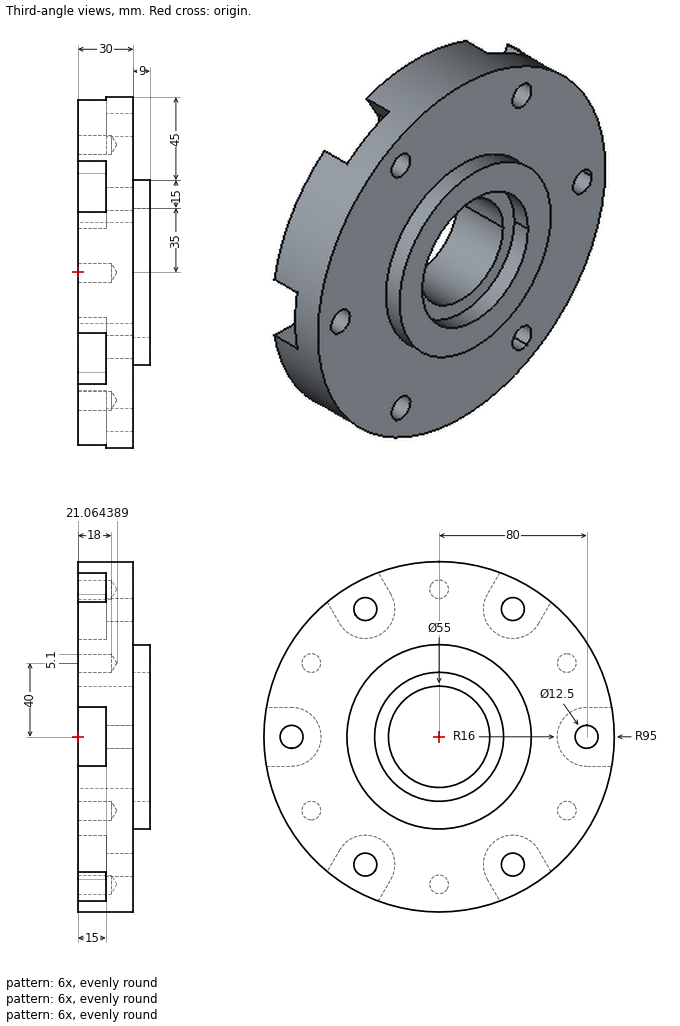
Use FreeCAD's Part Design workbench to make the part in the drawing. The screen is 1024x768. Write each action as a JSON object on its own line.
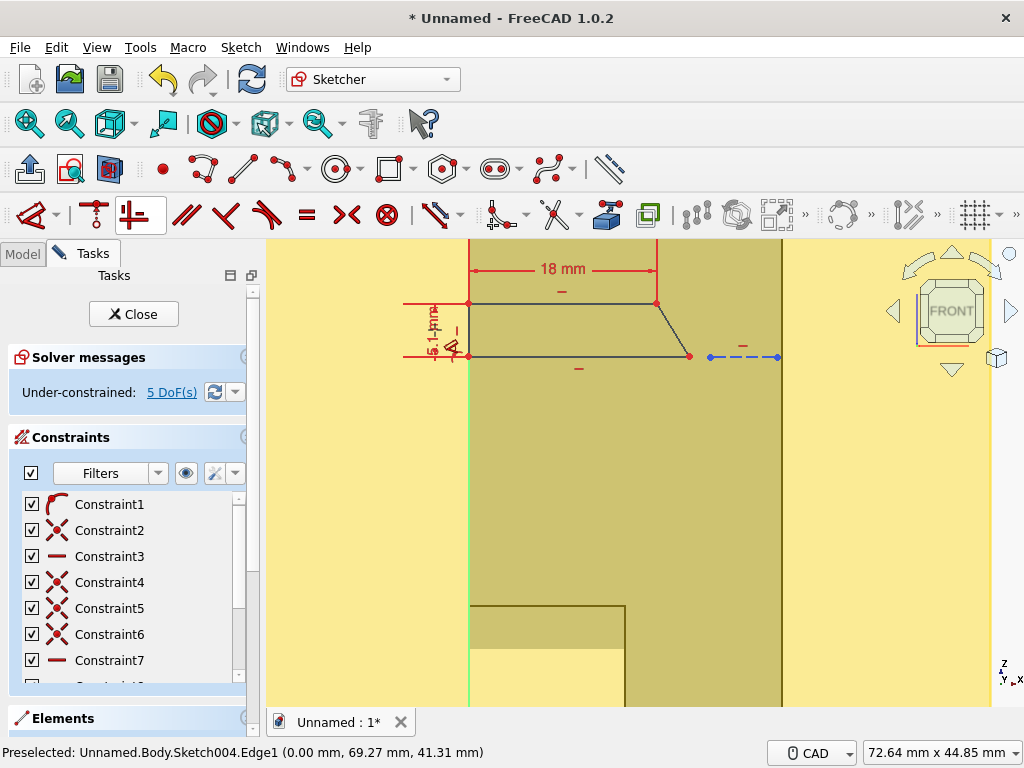
{"action": "left_click", "coordinate": [469, 357]}
{"action": "left_click", "coordinate": [435, 518]}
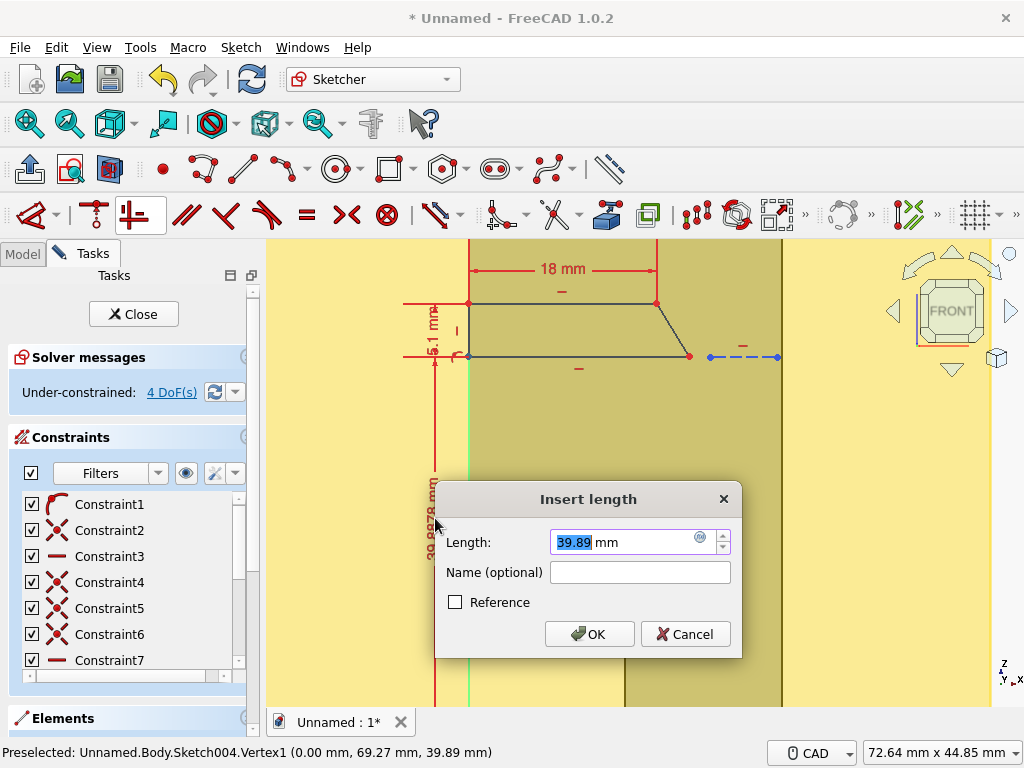
{"action": "type", "text": "40"}
{"action": "key", "text": "Return"}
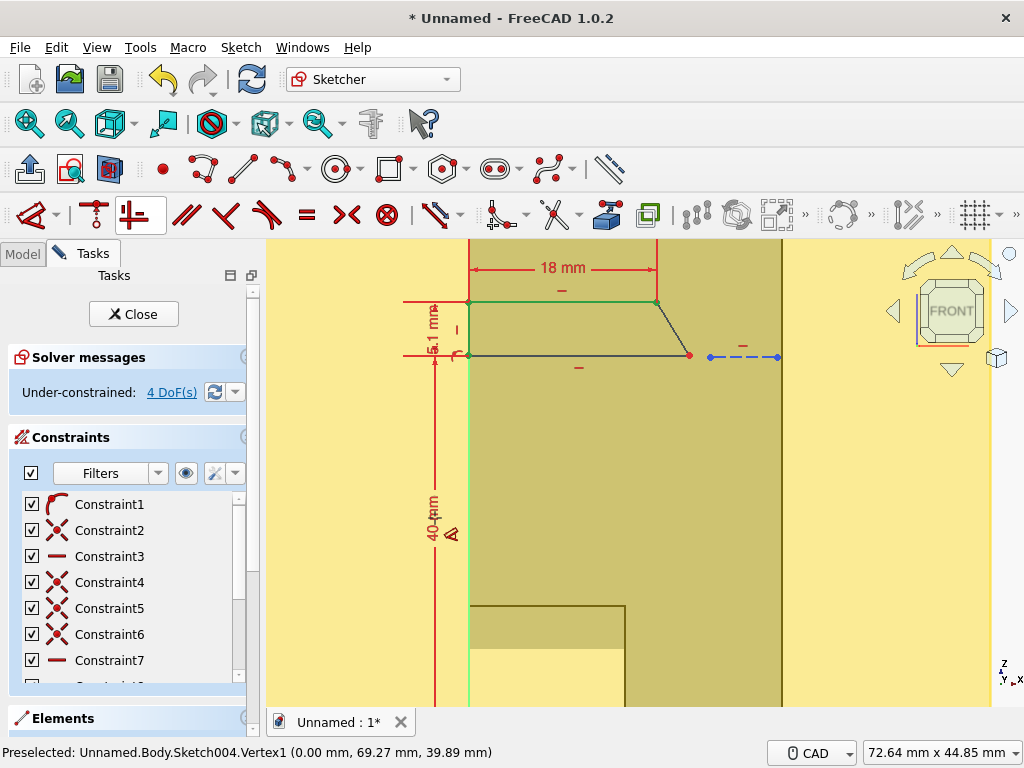
{"action": "left_click", "coordinate": [710, 357]}
{"action": "left_click", "coordinate": [435, 444]}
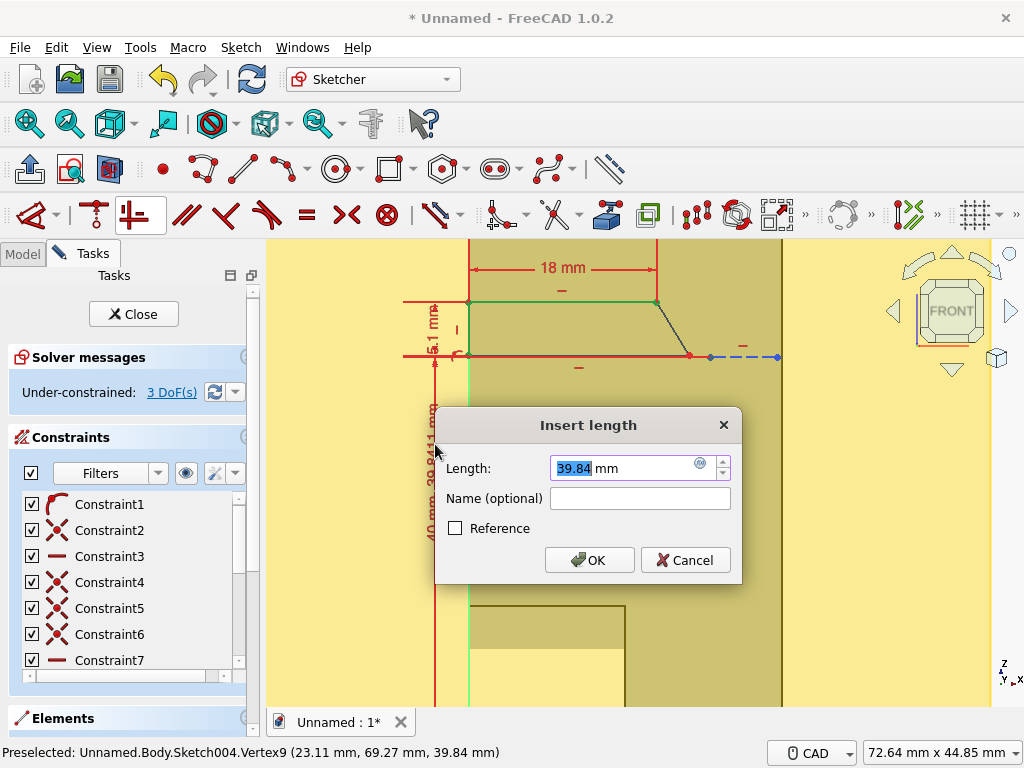
{"action": "type", "text": "40"}
{"action": "key", "text": "Return"}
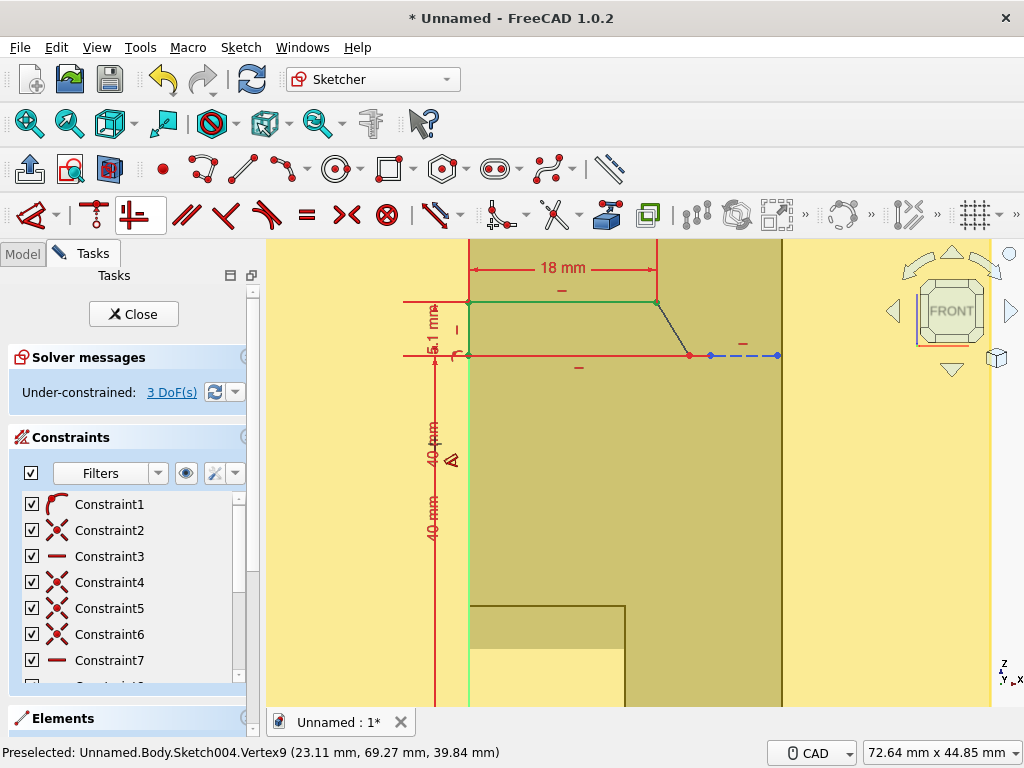
{"action": "left_click", "coordinate": [623, 356]}
{"action": "left_click", "coordinate": [579, 322]}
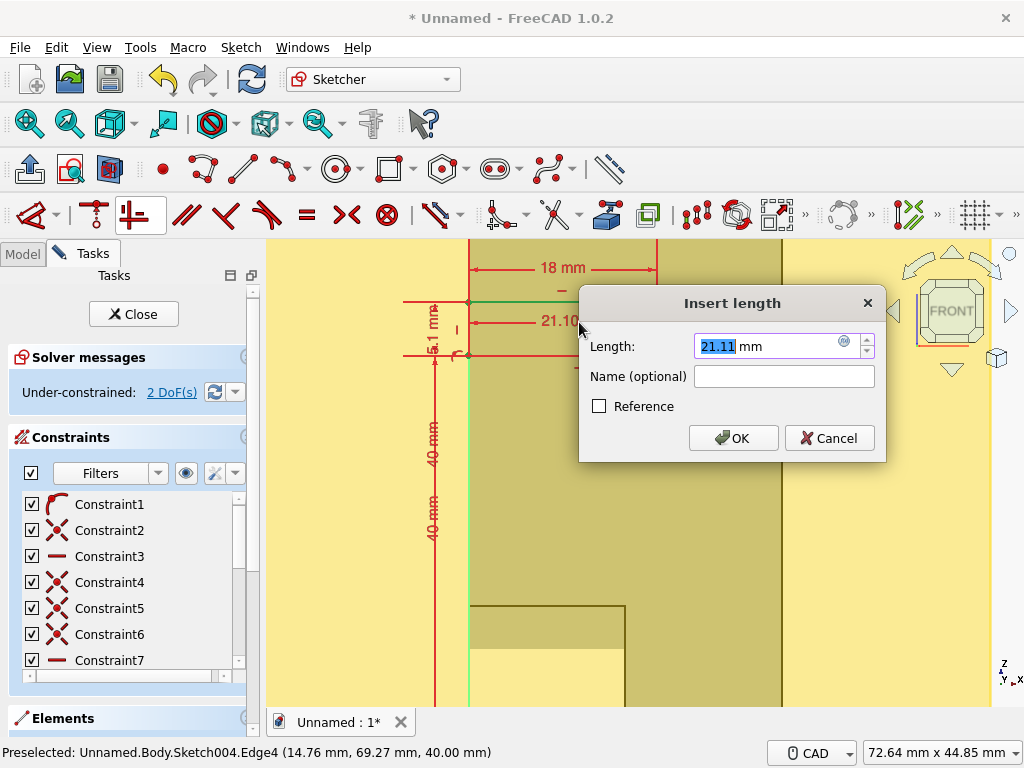
{"action": "type", "text": "21.064389"}
{"action": "key", "text": "Return"}
{"action": "key", "text": "Escape"}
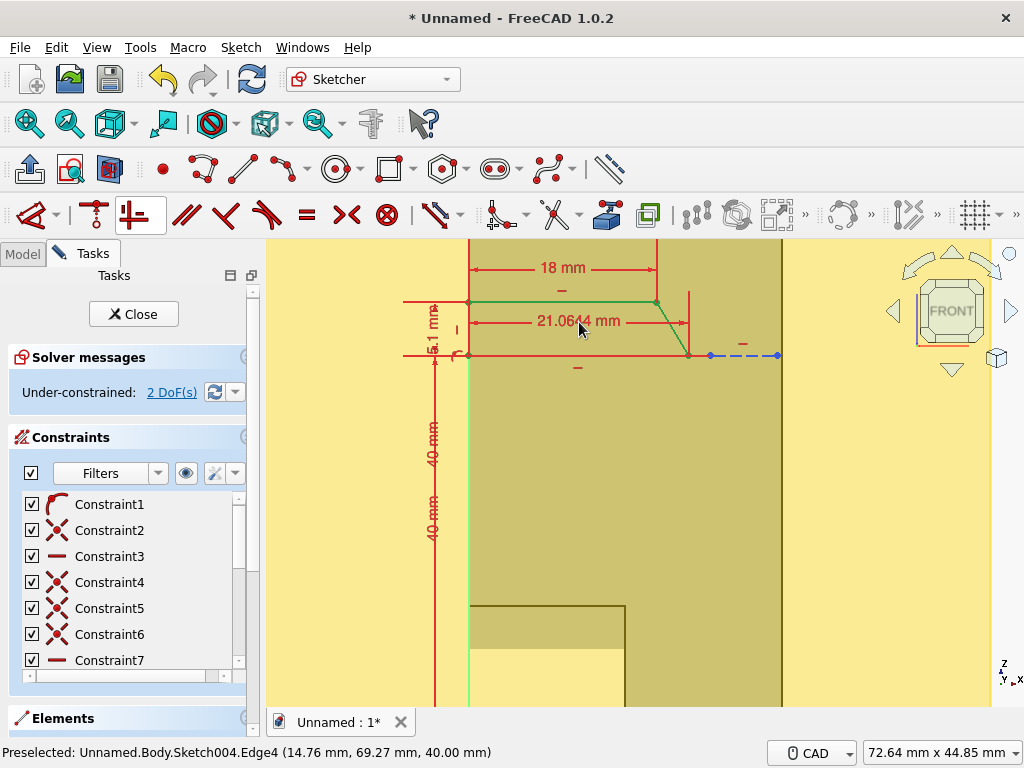
{"action": "left_click", "coordinate": [134, 314]}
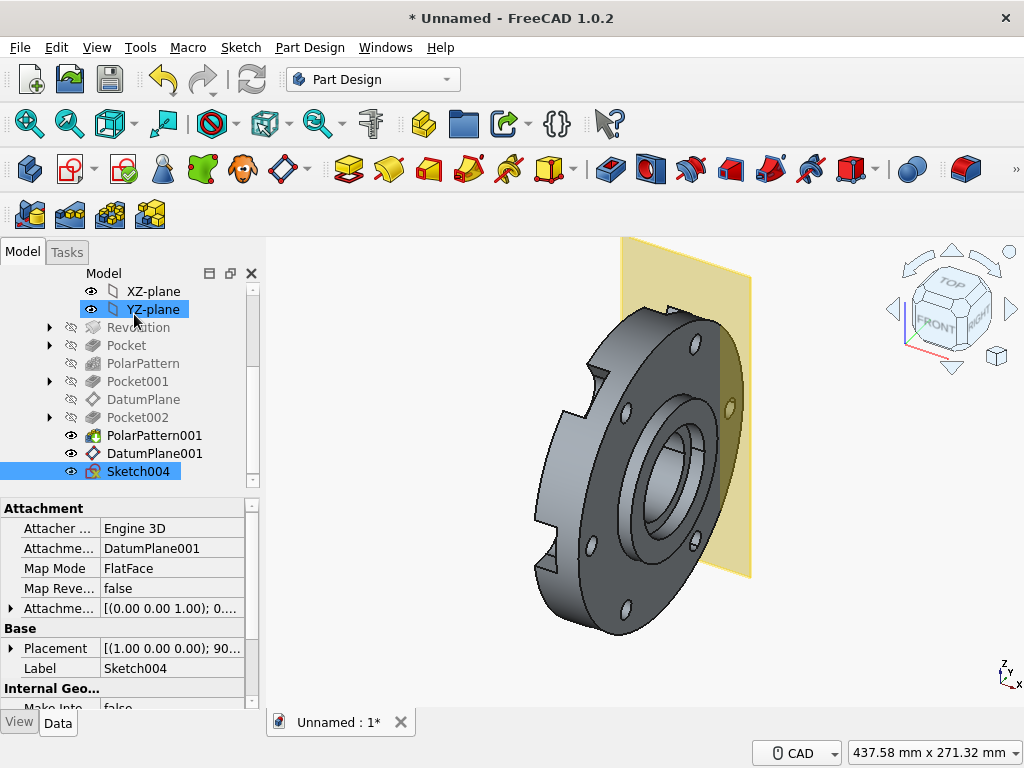
{"action": "left_click", "coordinate": [692, 170]}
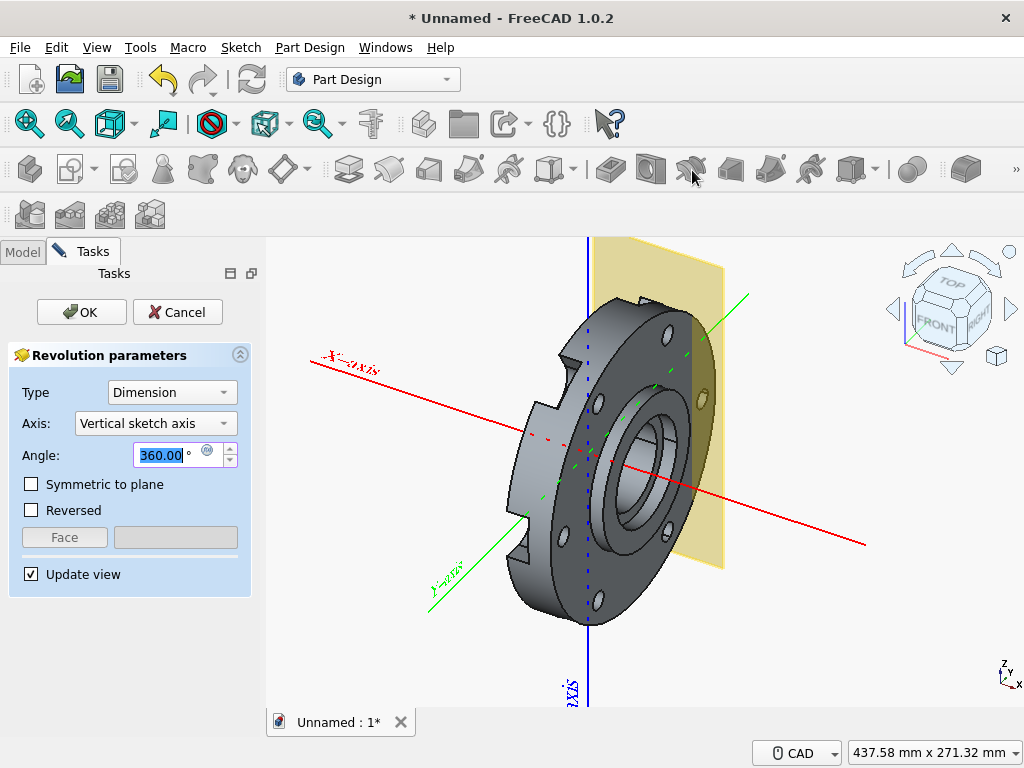
{"action": "left_click", "coordinate": [156, 424]}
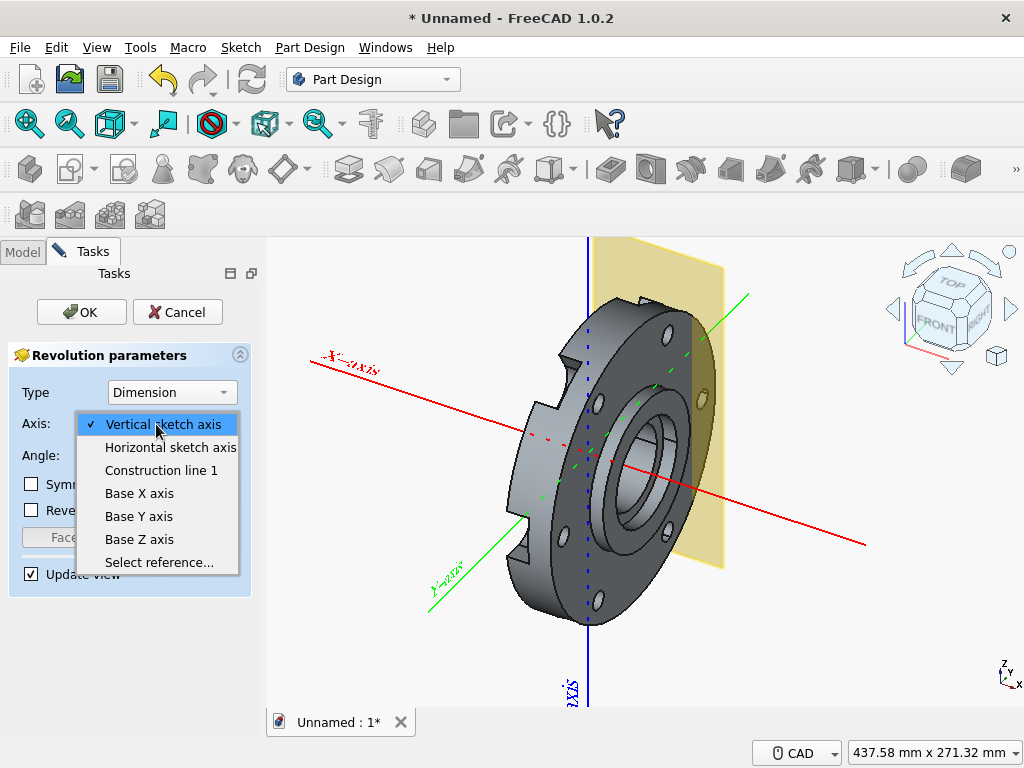
{"action": "left_click", "coordinate": [156, 470]}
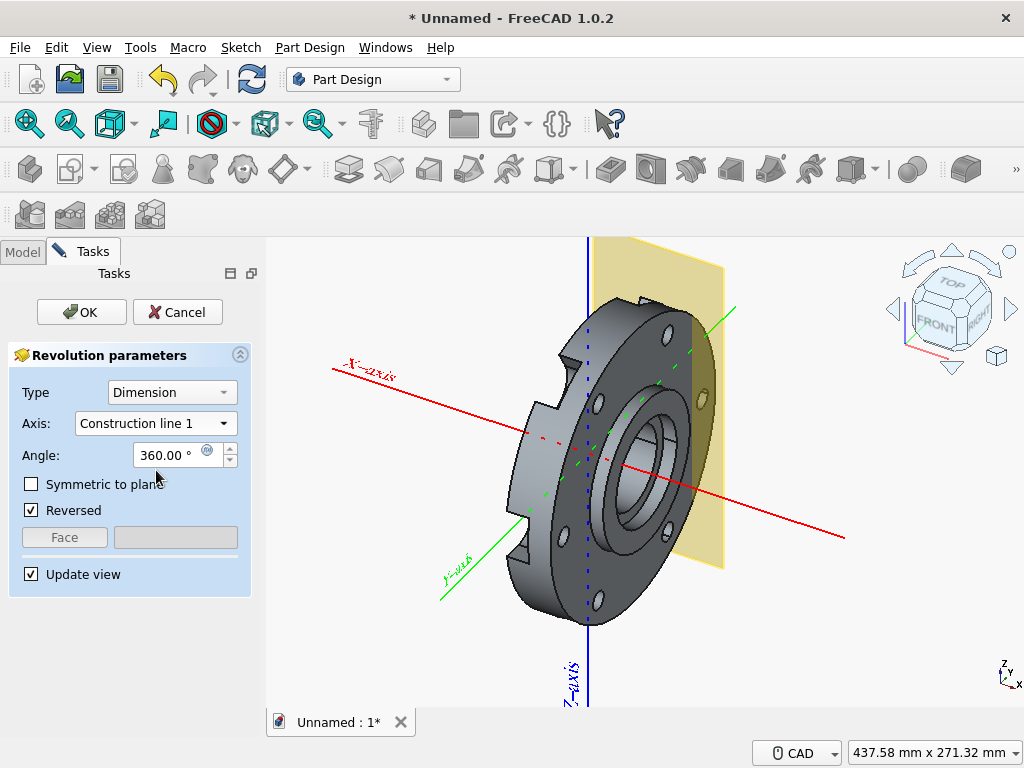
{"action": "left_click", "coordinate": [82, 312]}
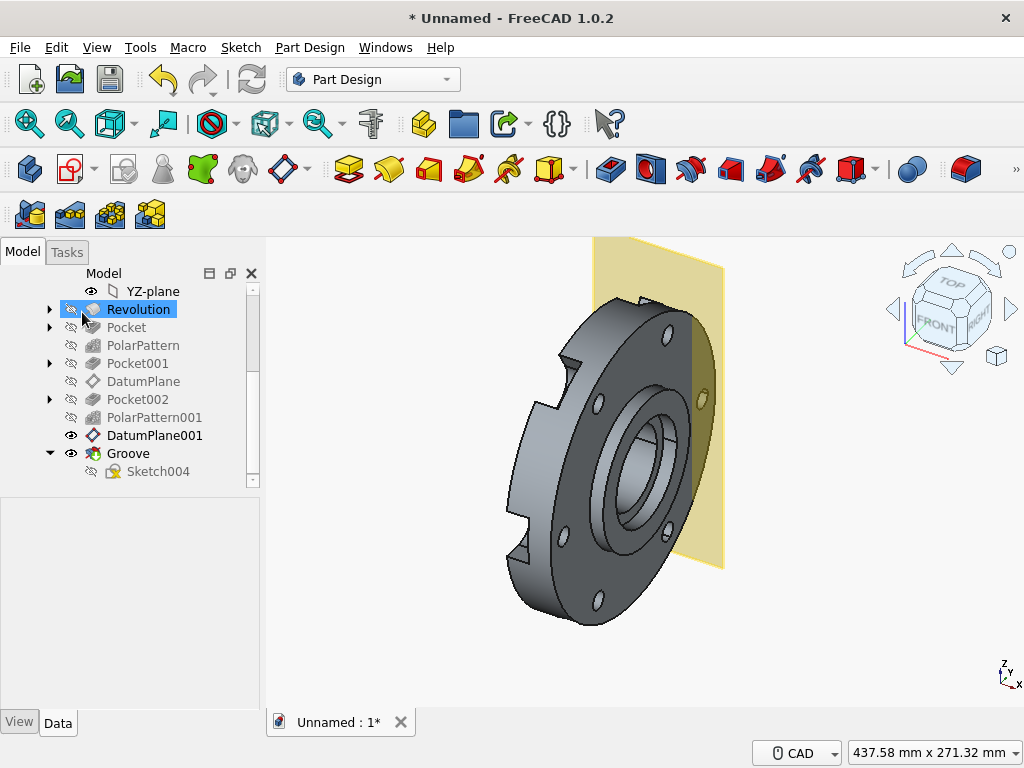
{"action": "left_click", "coordinate": [116, 435]}
{"action": "key", "text": "space"}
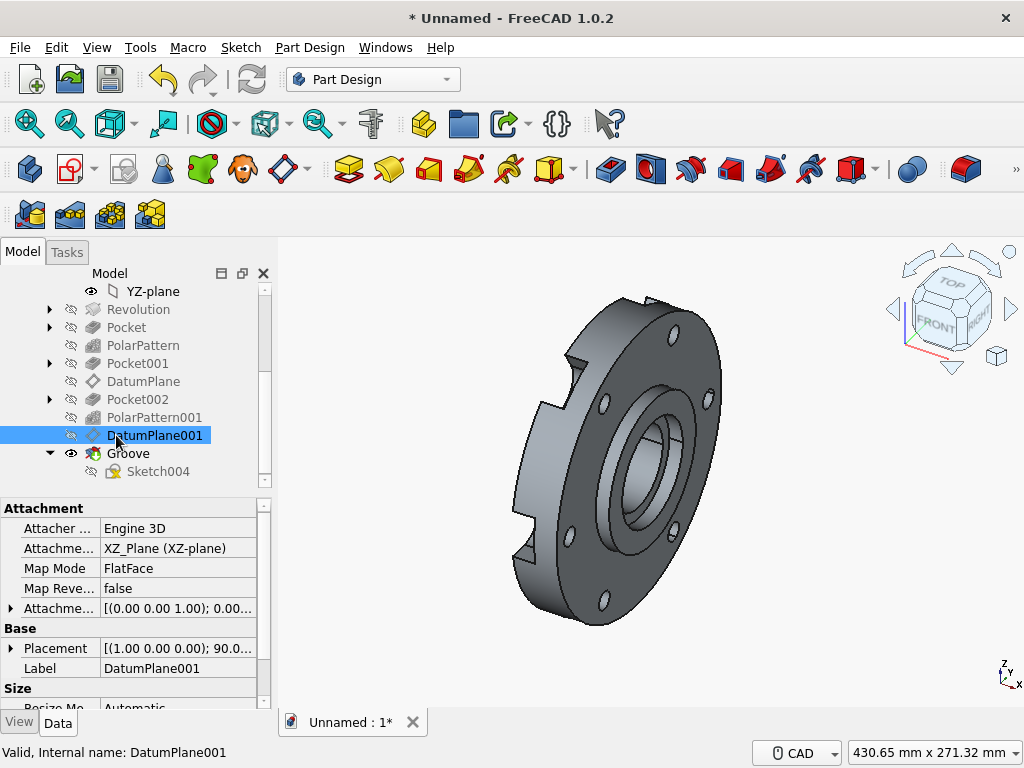
{"action": "left_click", "coordinate": [30, 124]}